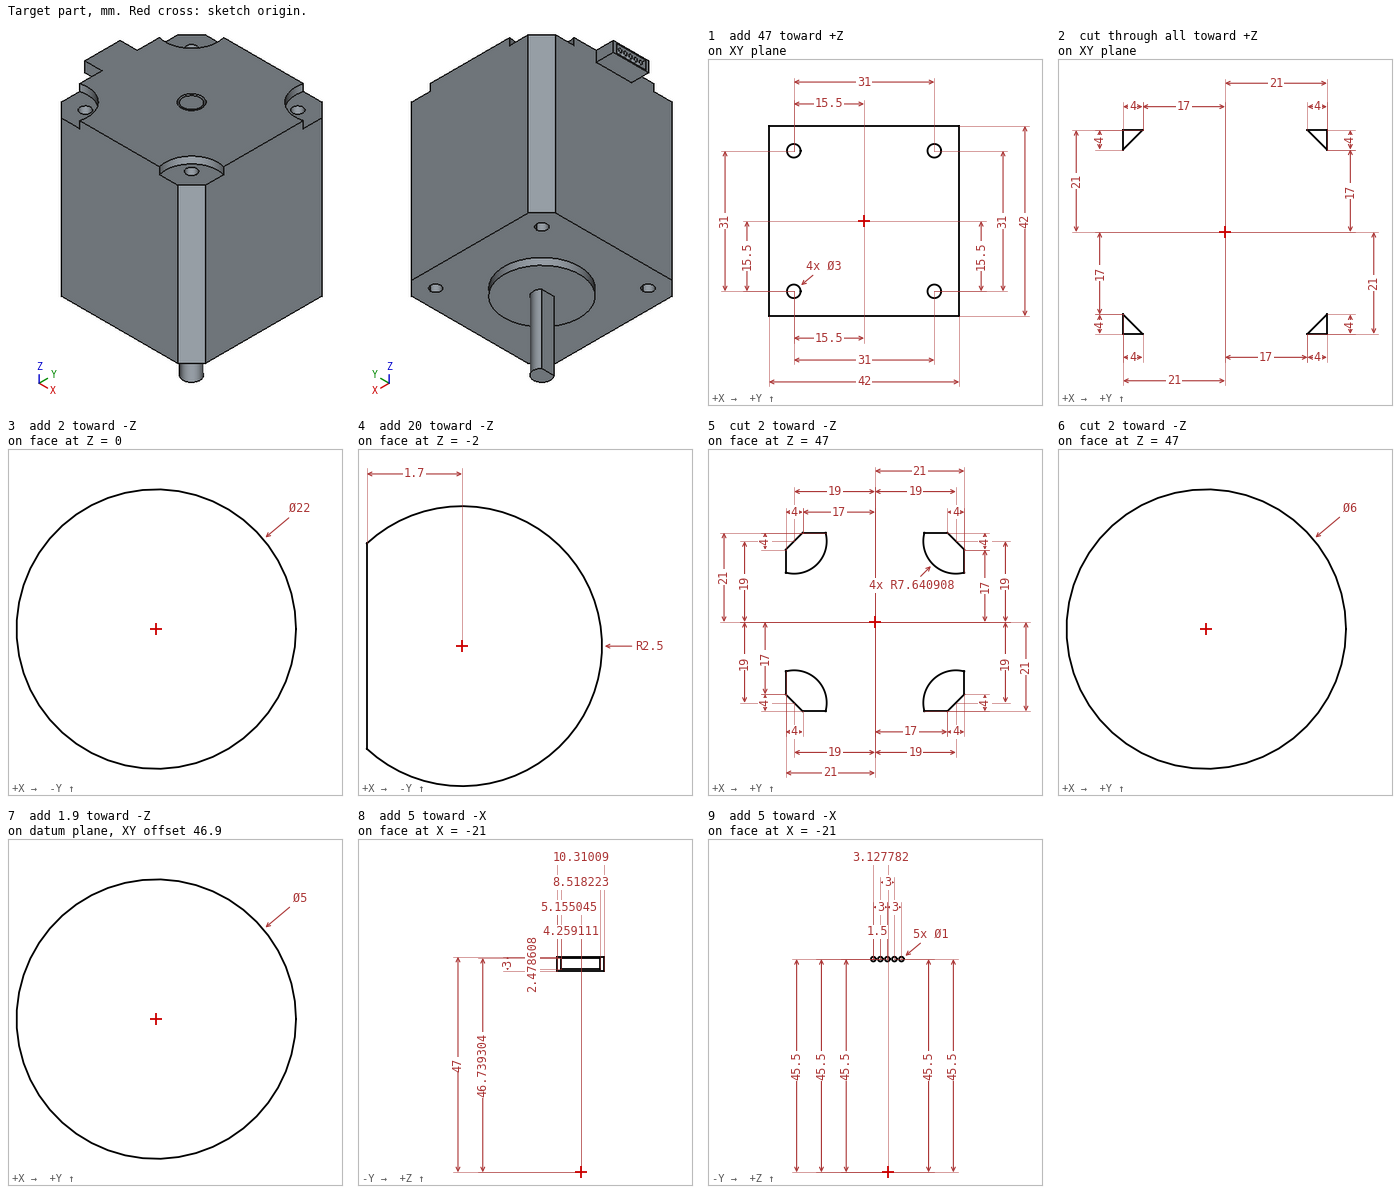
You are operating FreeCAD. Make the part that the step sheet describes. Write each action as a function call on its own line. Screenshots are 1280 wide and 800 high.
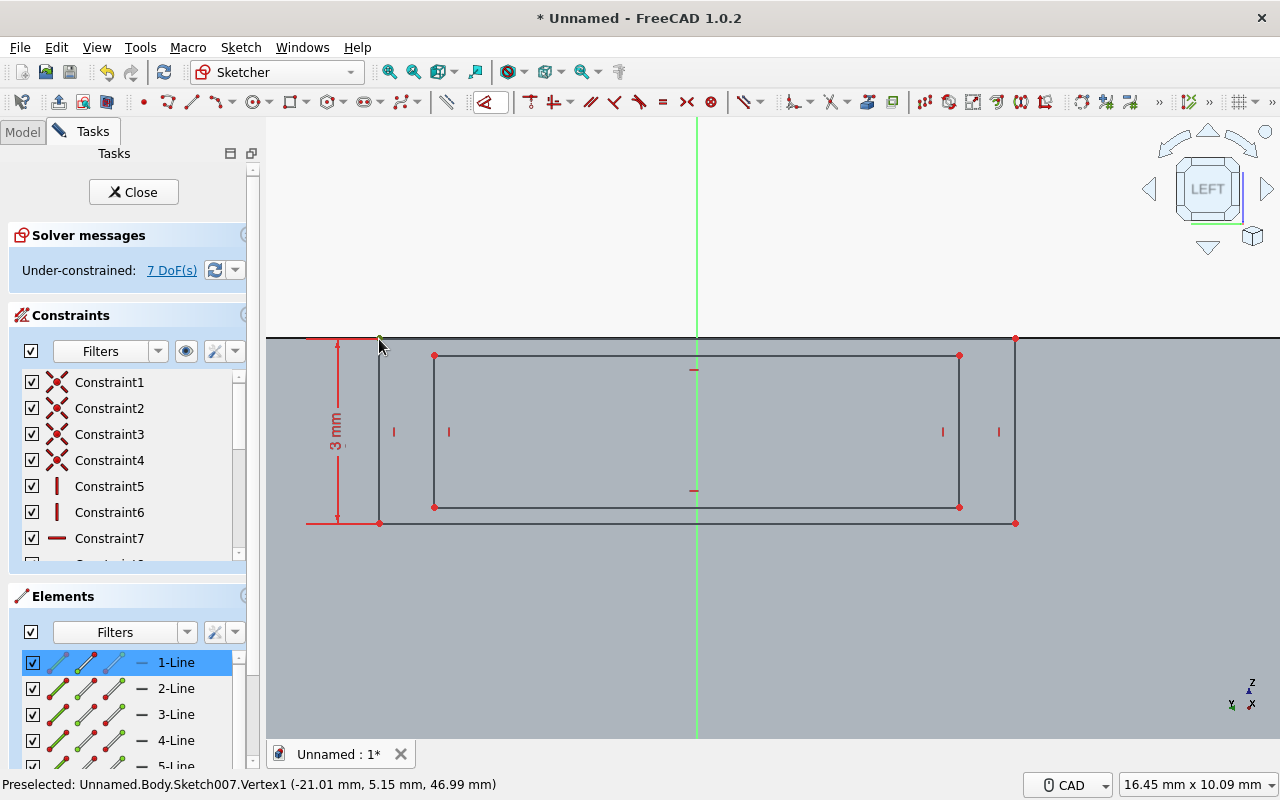
key(i)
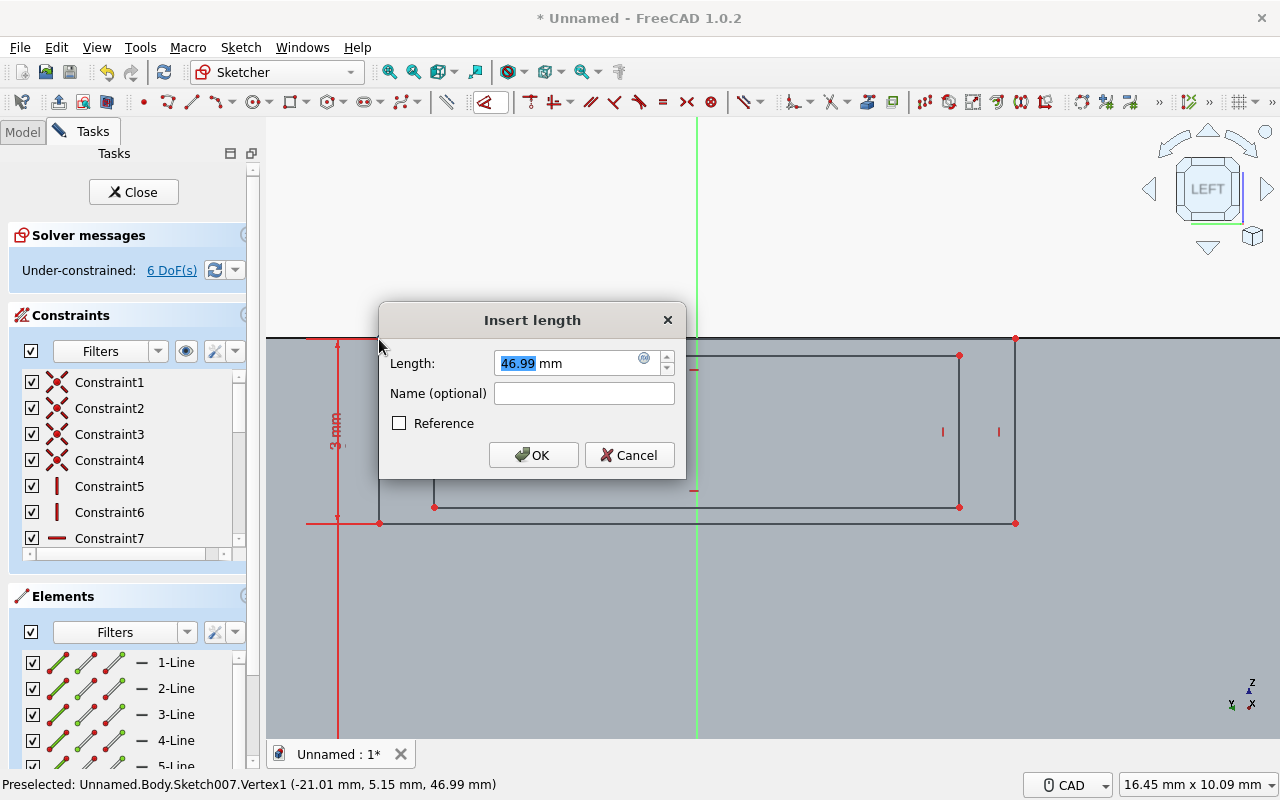
text(47)
key(Return)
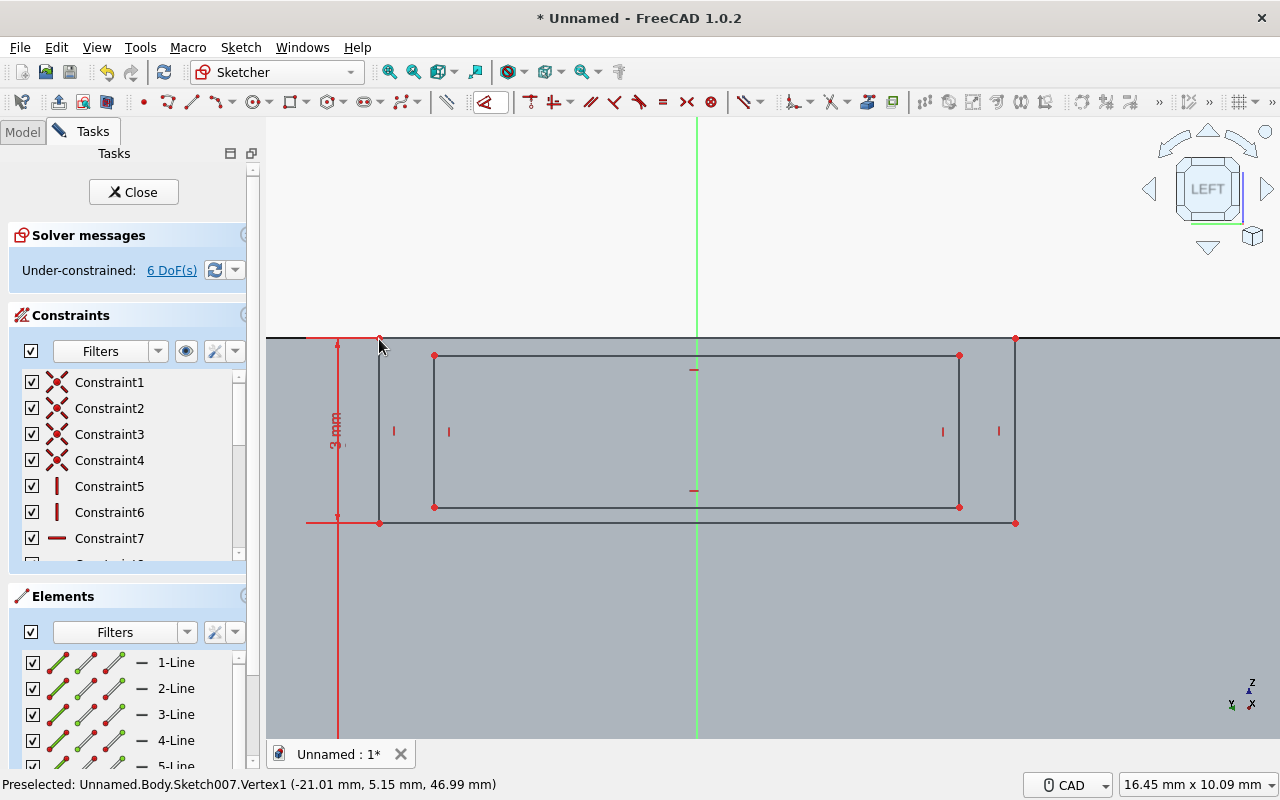
click(570, 523)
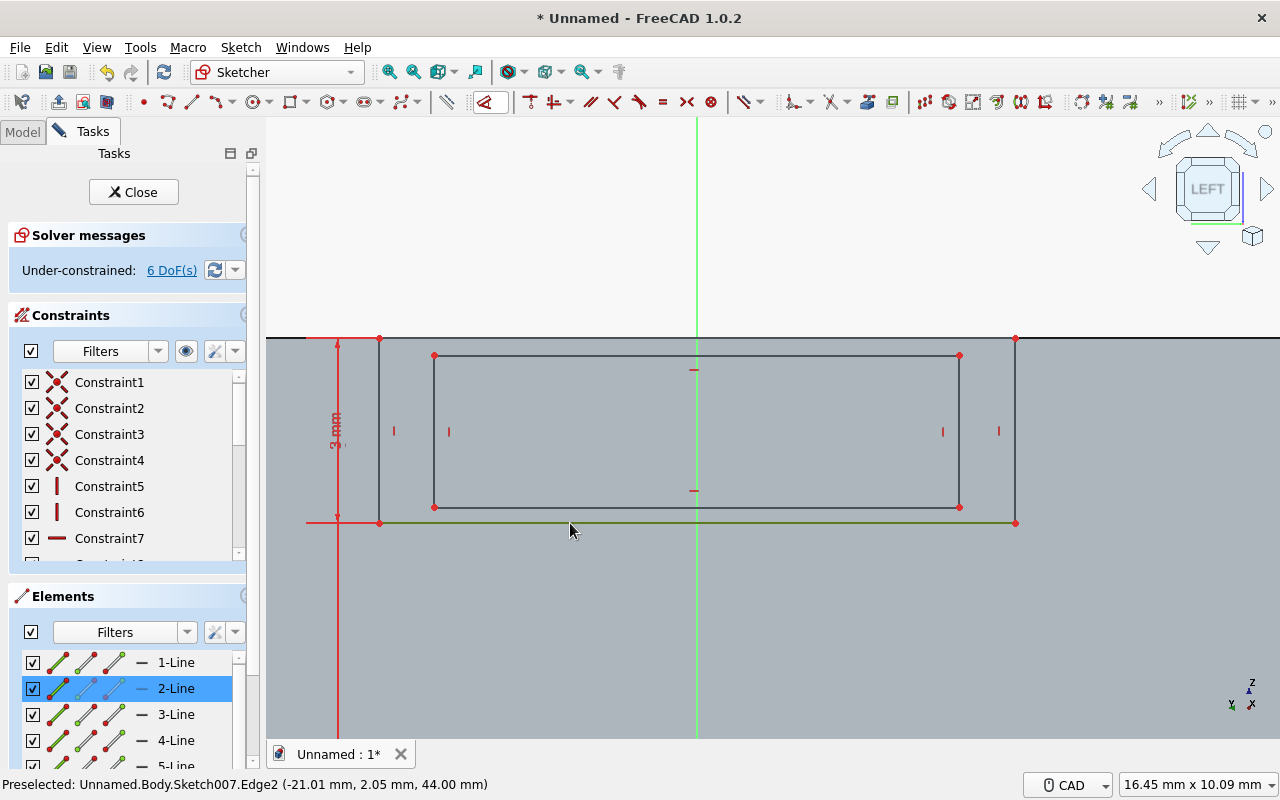
click(502, 102)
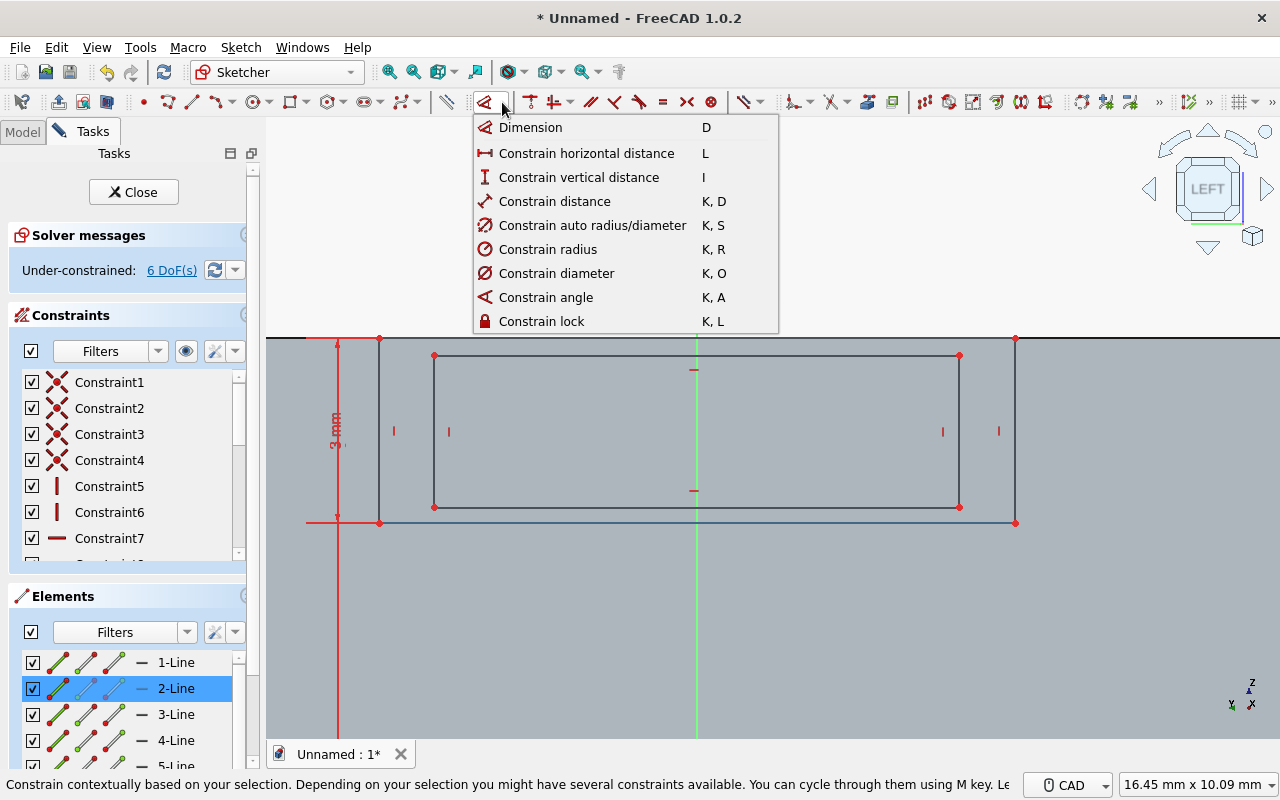
click(626, 153)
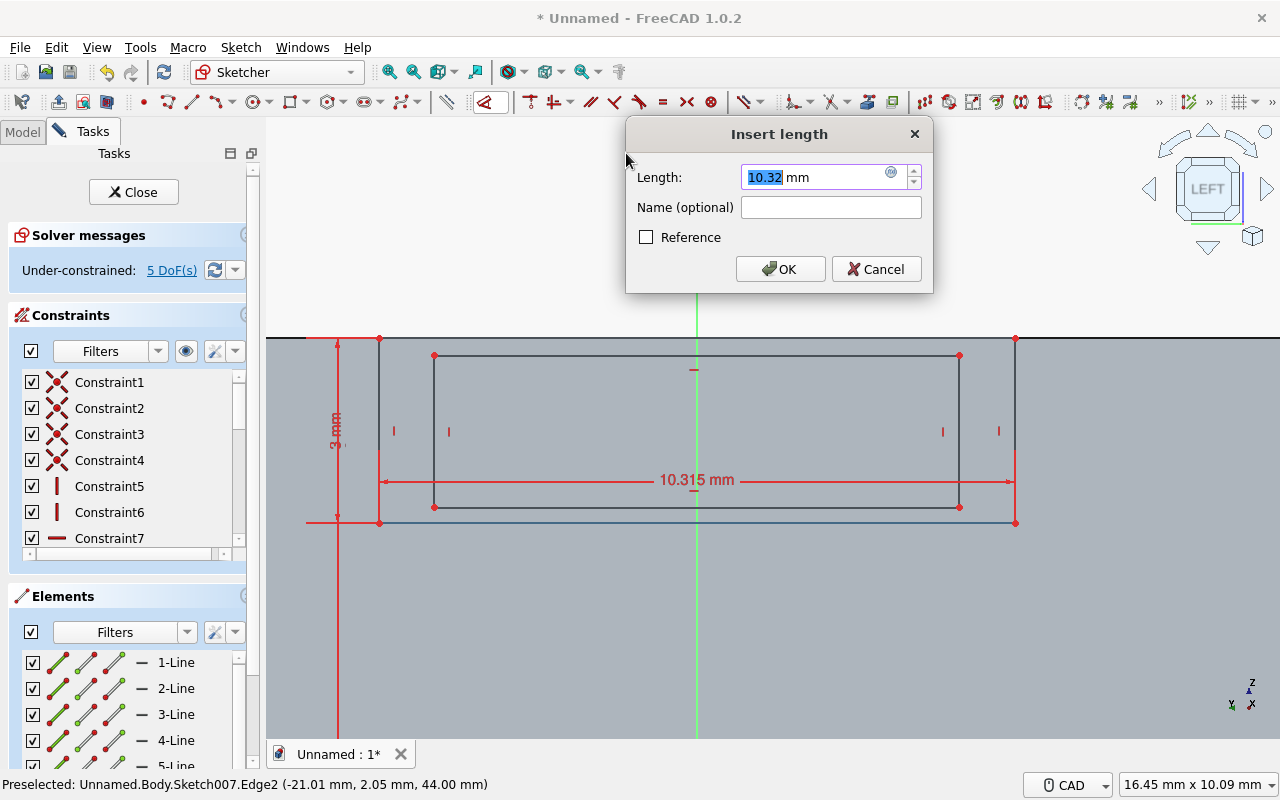
text(10.31009)
key(Return)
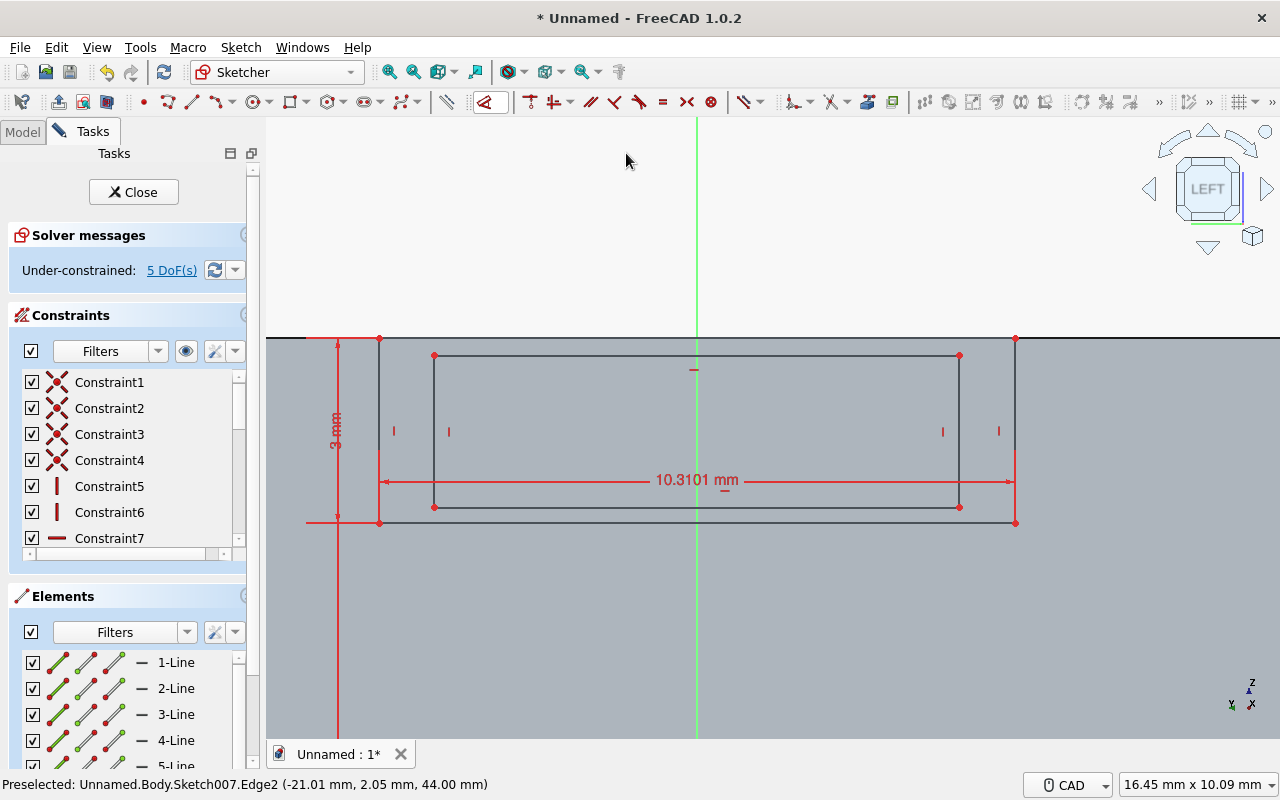
click(434, 402)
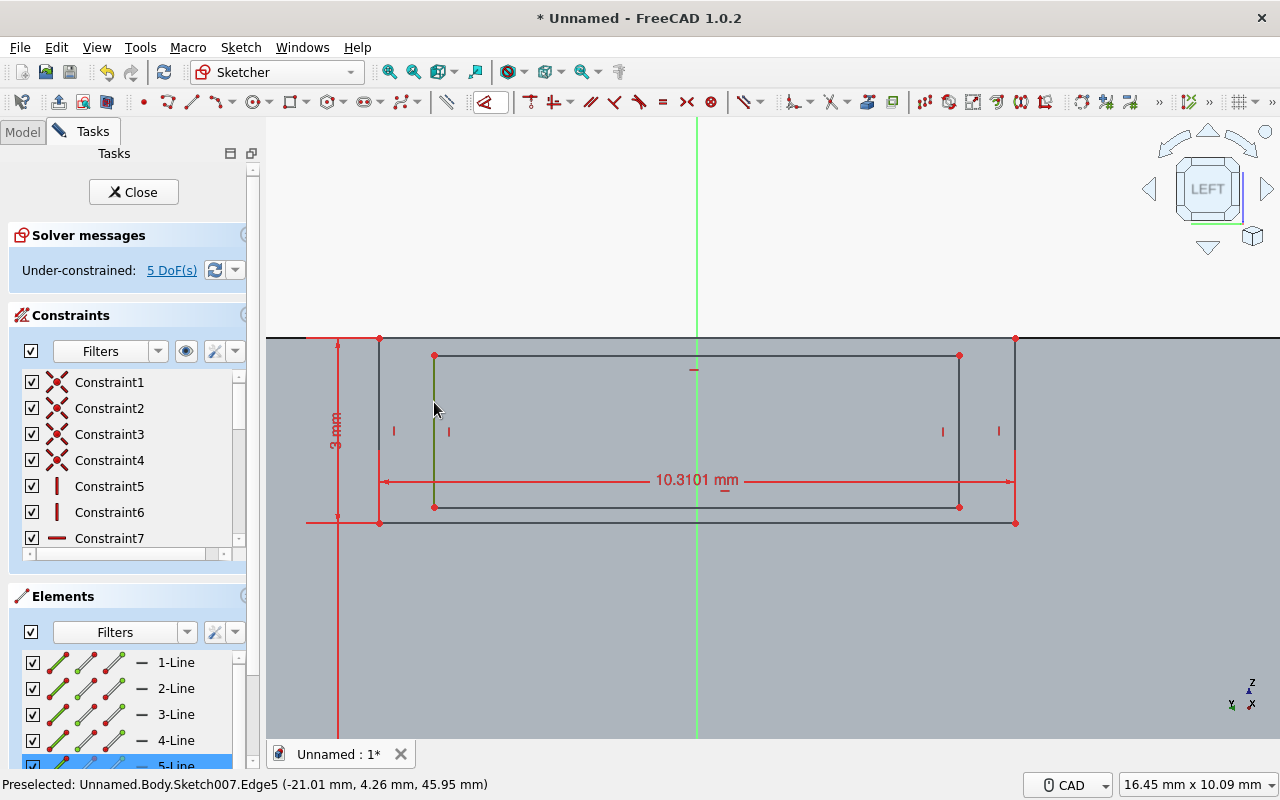
key(i)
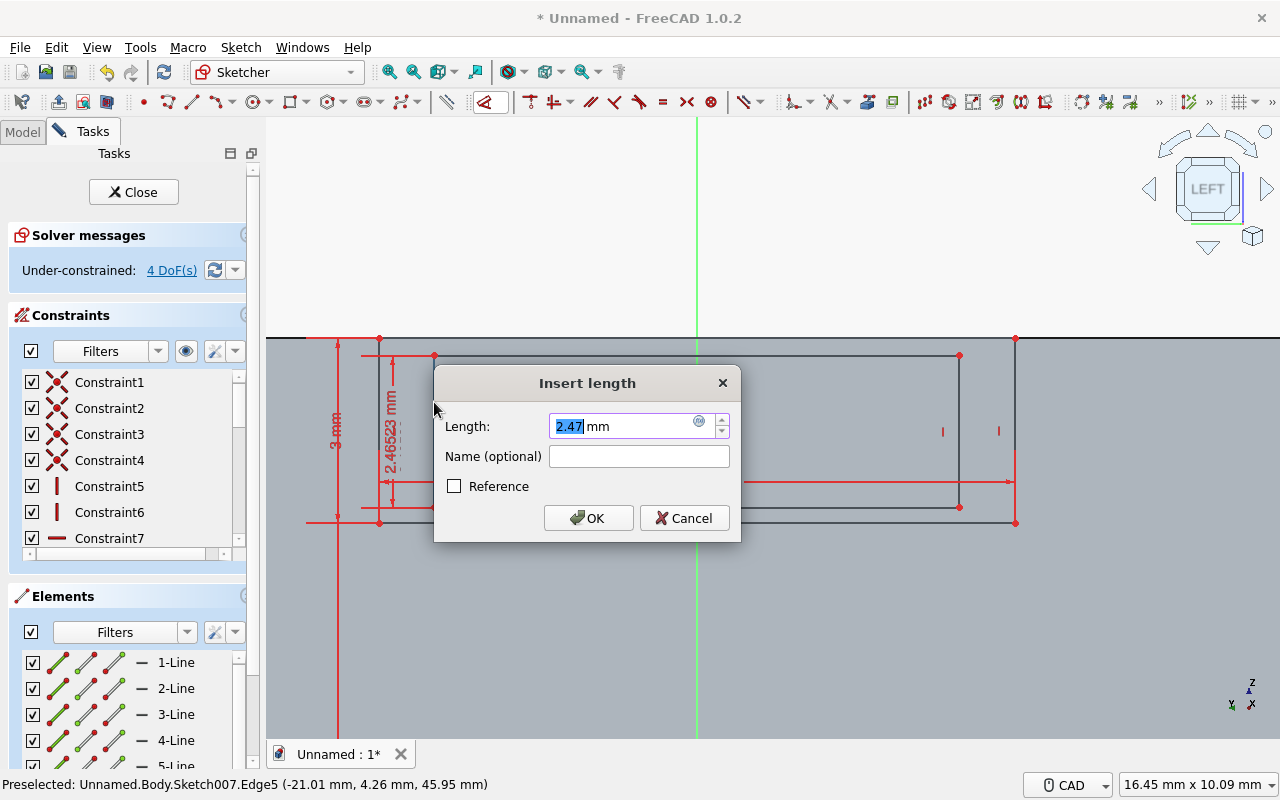
text(2.478608)
key(Return)